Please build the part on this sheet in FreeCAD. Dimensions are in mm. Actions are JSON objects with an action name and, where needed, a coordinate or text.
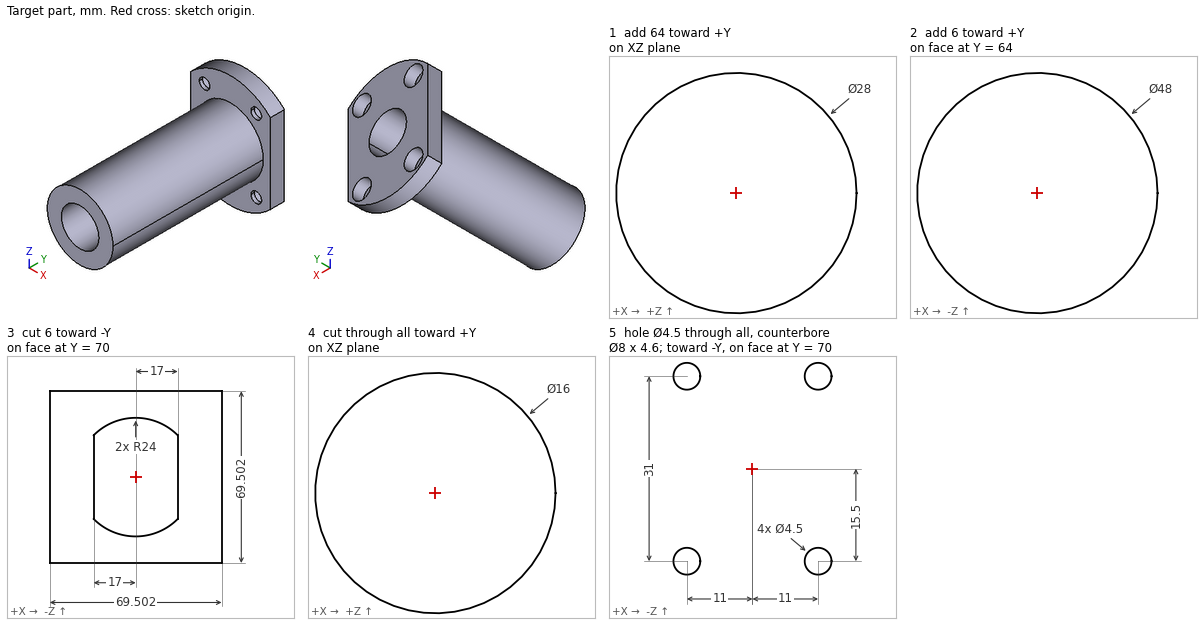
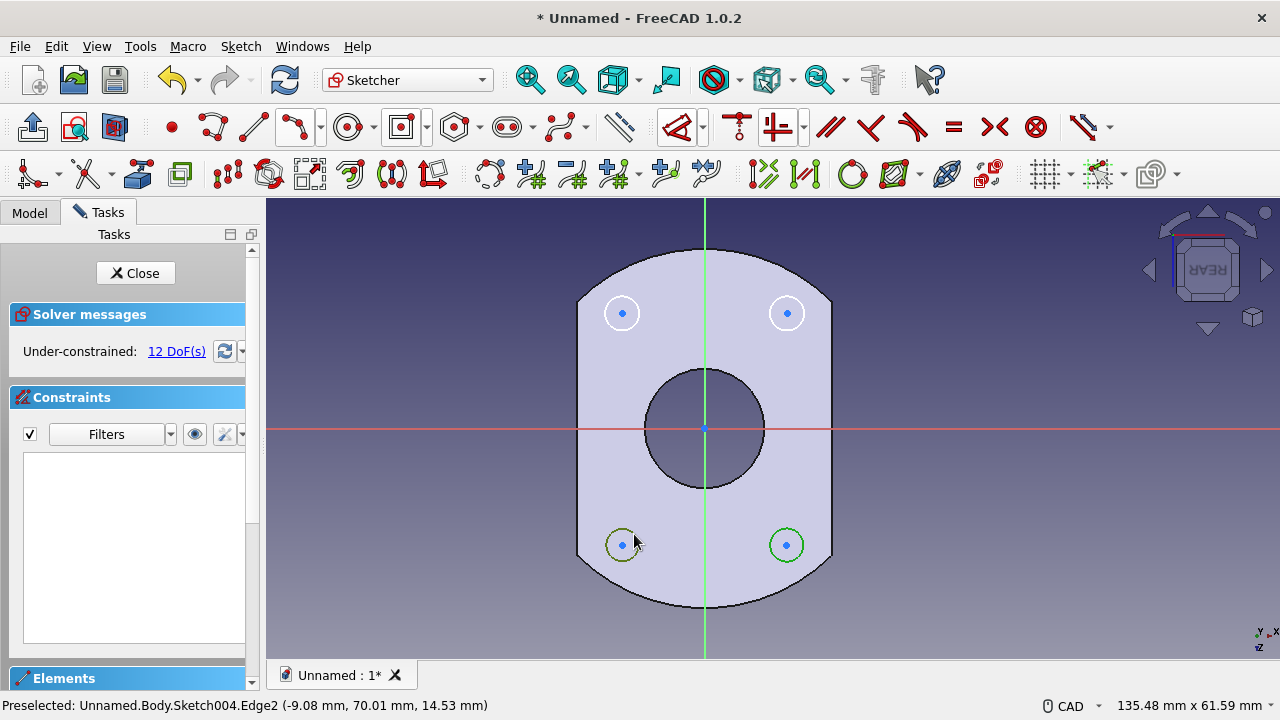
{"action": "left_click", "coordinate": [634, 301]}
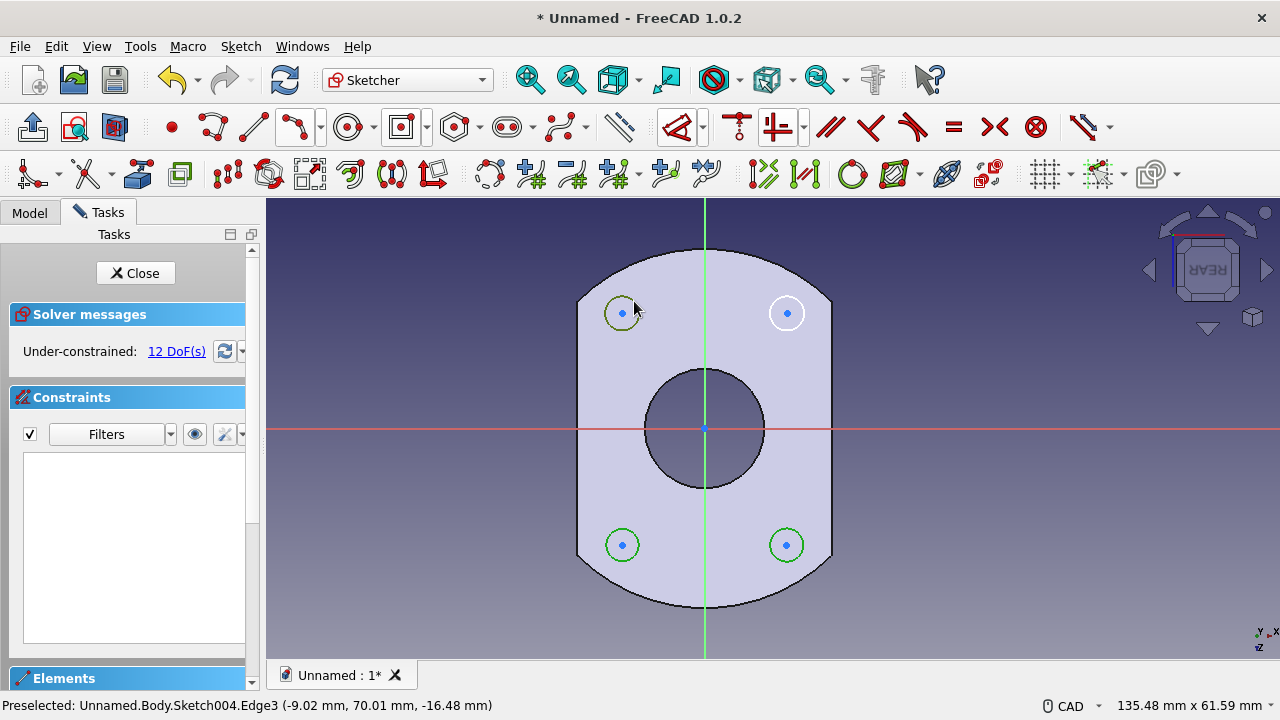
{"action": "left_click", "coordinate": [799, 301]}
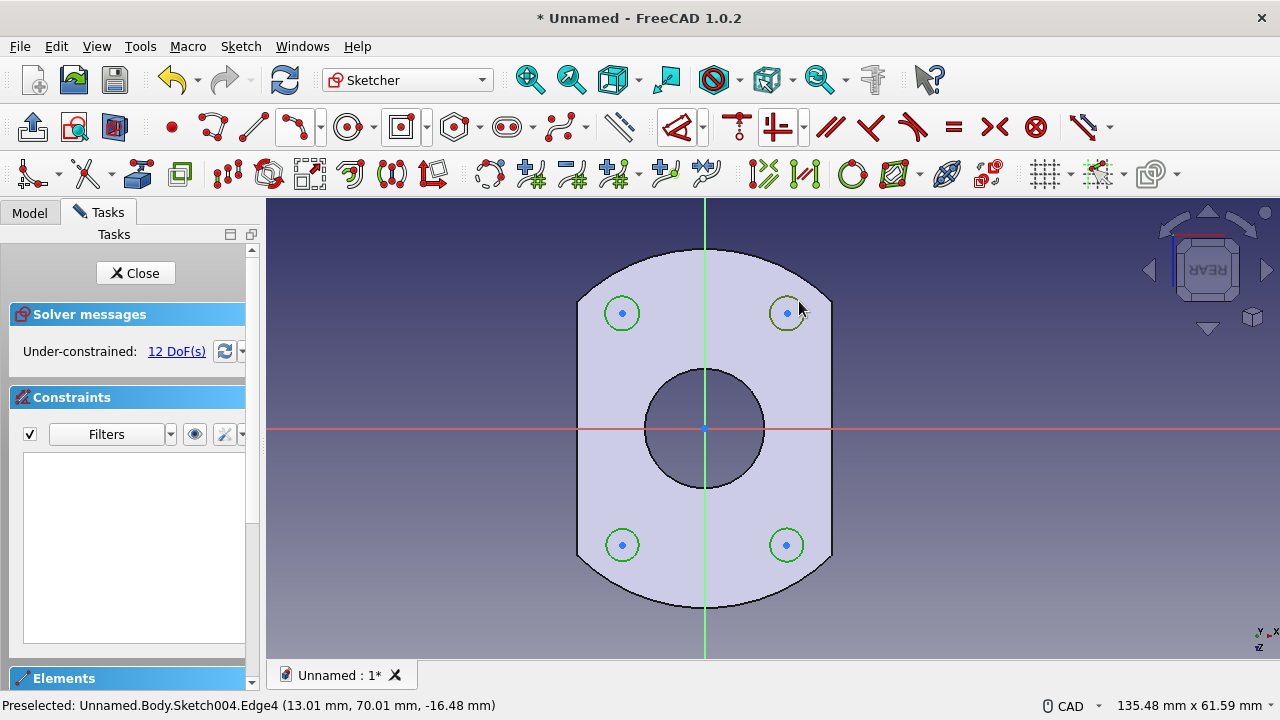
{"action": "left_click", "coordinate": [954, 128]}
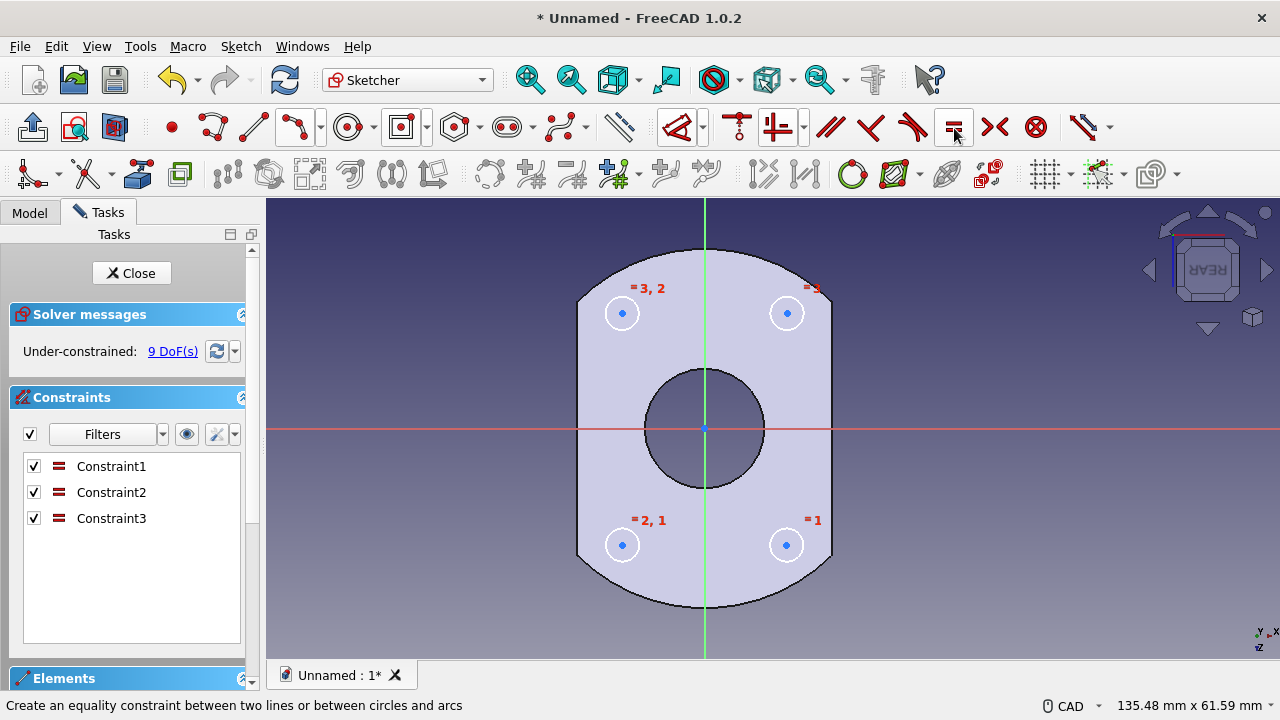
{"action": "left_click", "coordinate": [787, 545]}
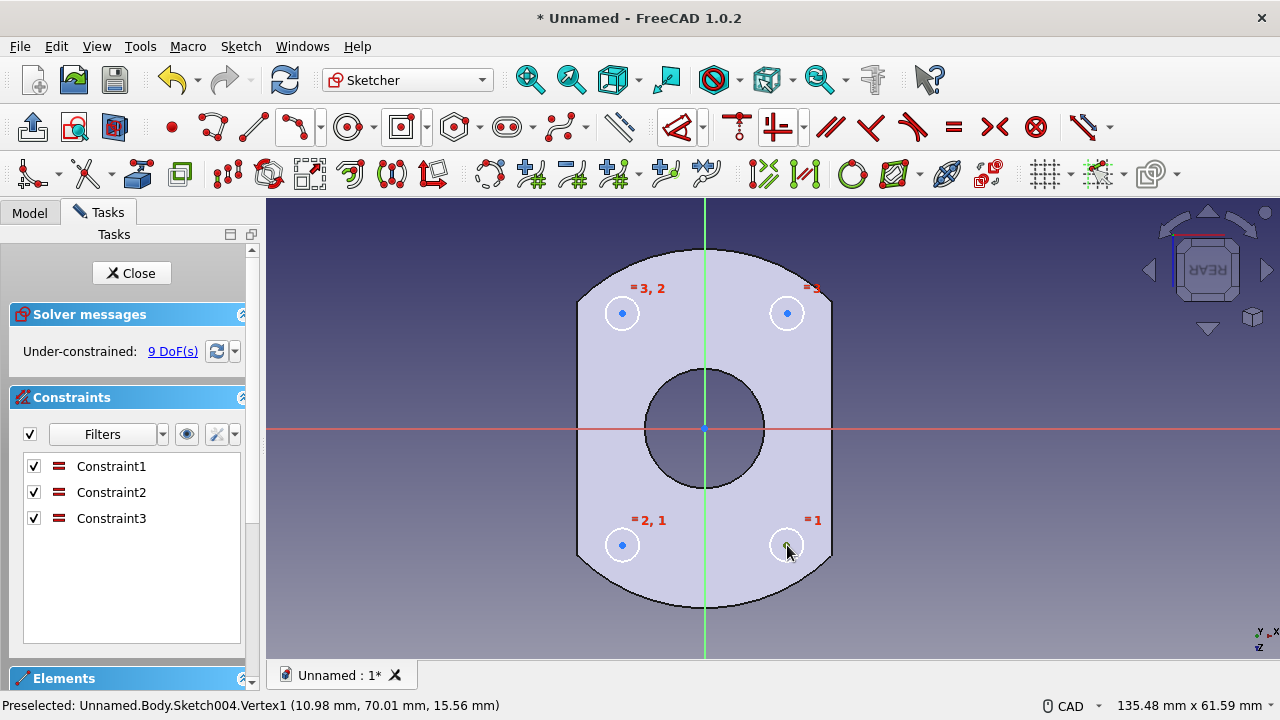
{"action": "left_click", "coordinate": [622, 545]}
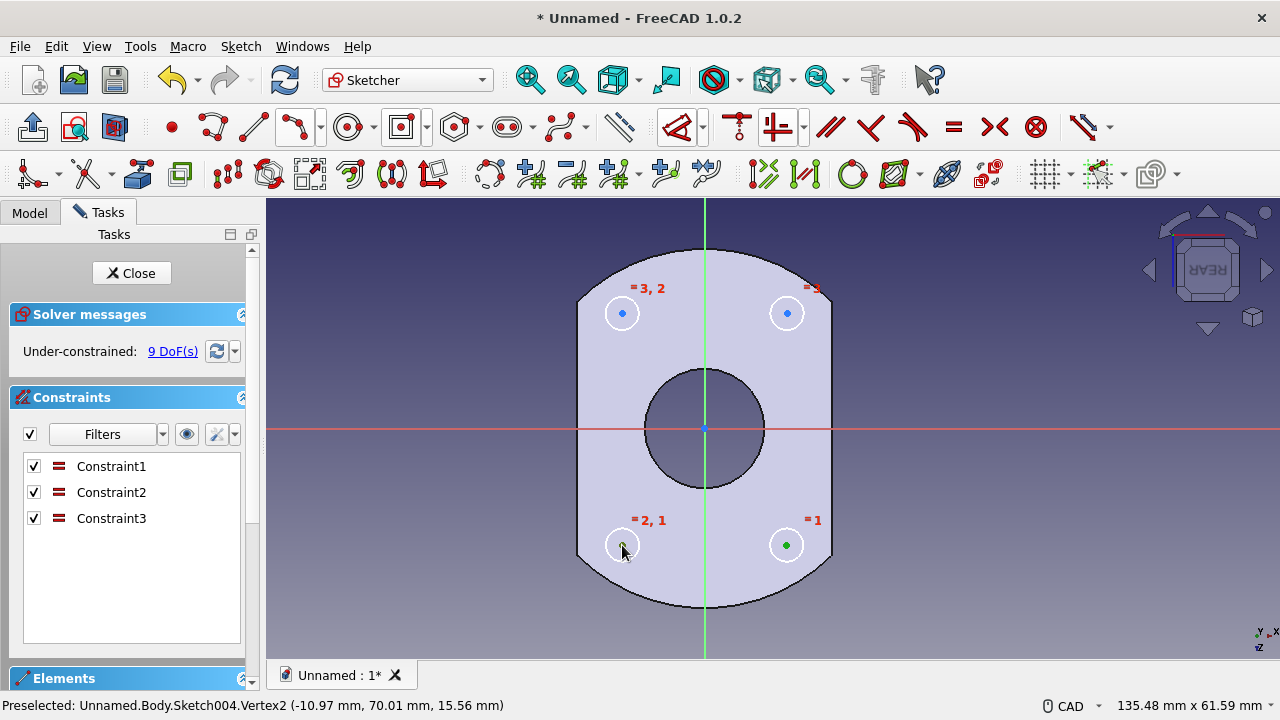
{"action": "key", "text": "h"}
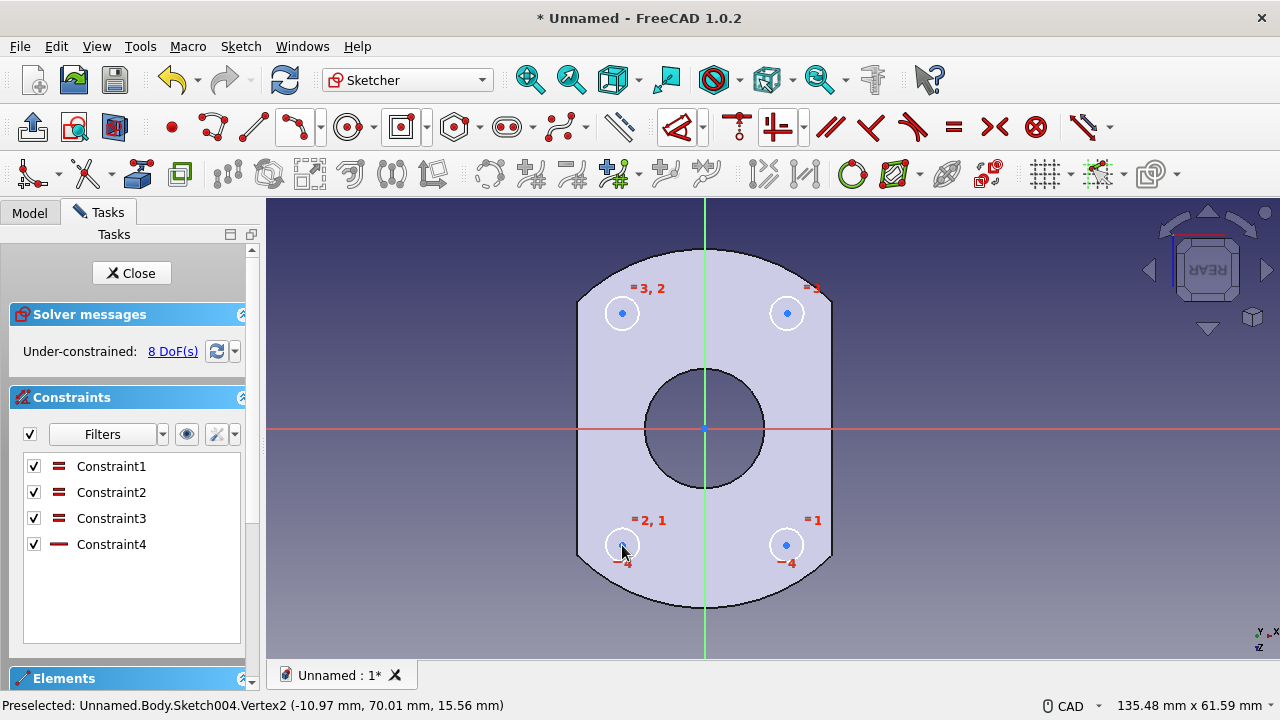
{"action": "left_click", "coordinate": [622, 545]}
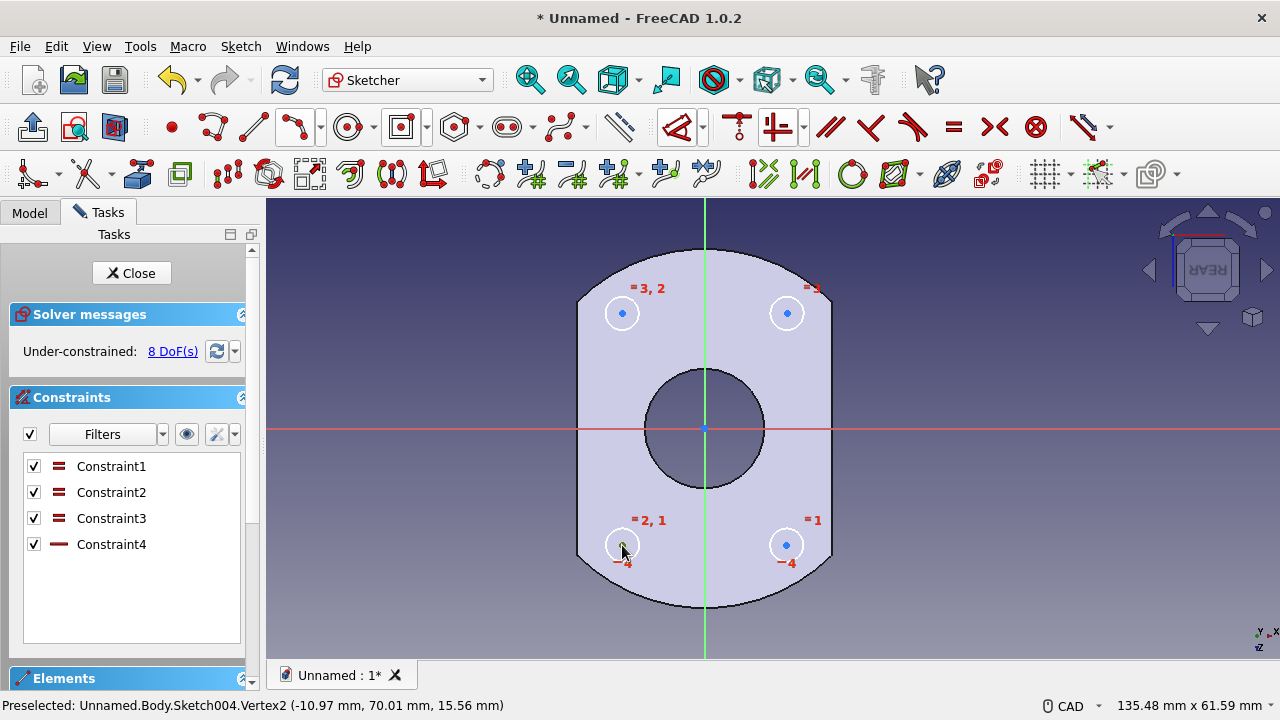
{"action": "left_click", "coordinate": [622, 313]}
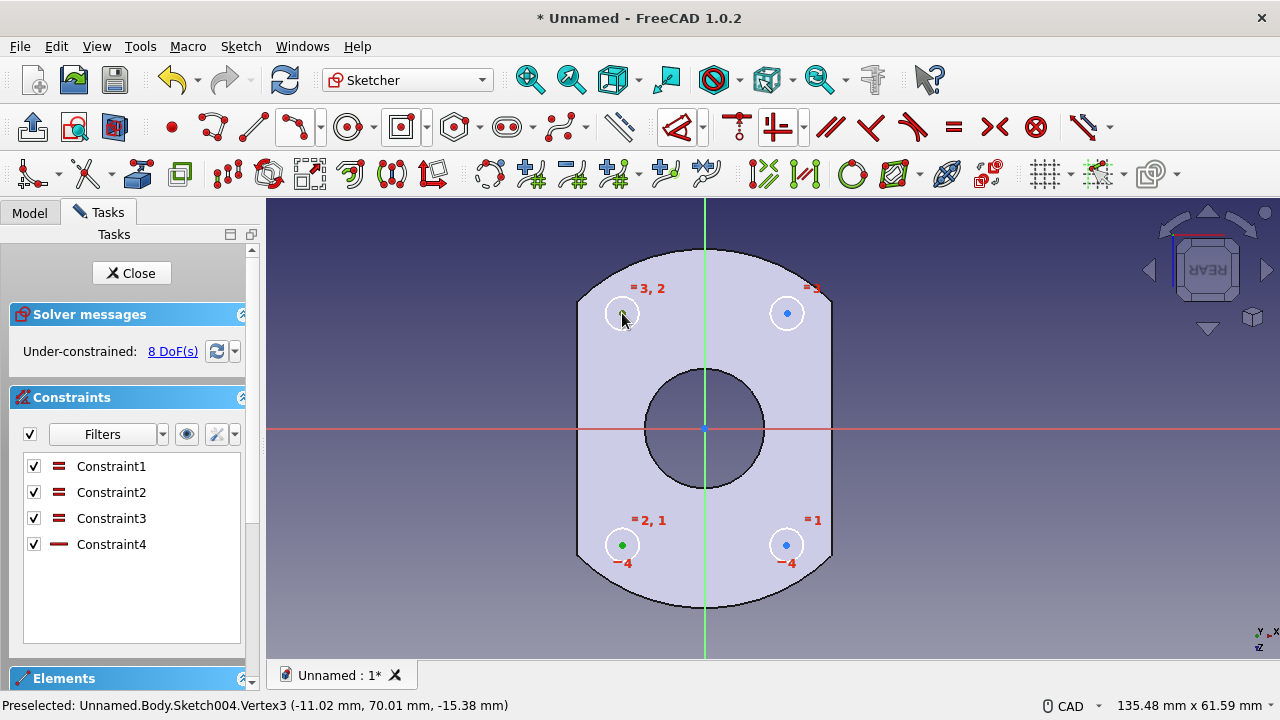
{"action": "key", "text": "v"}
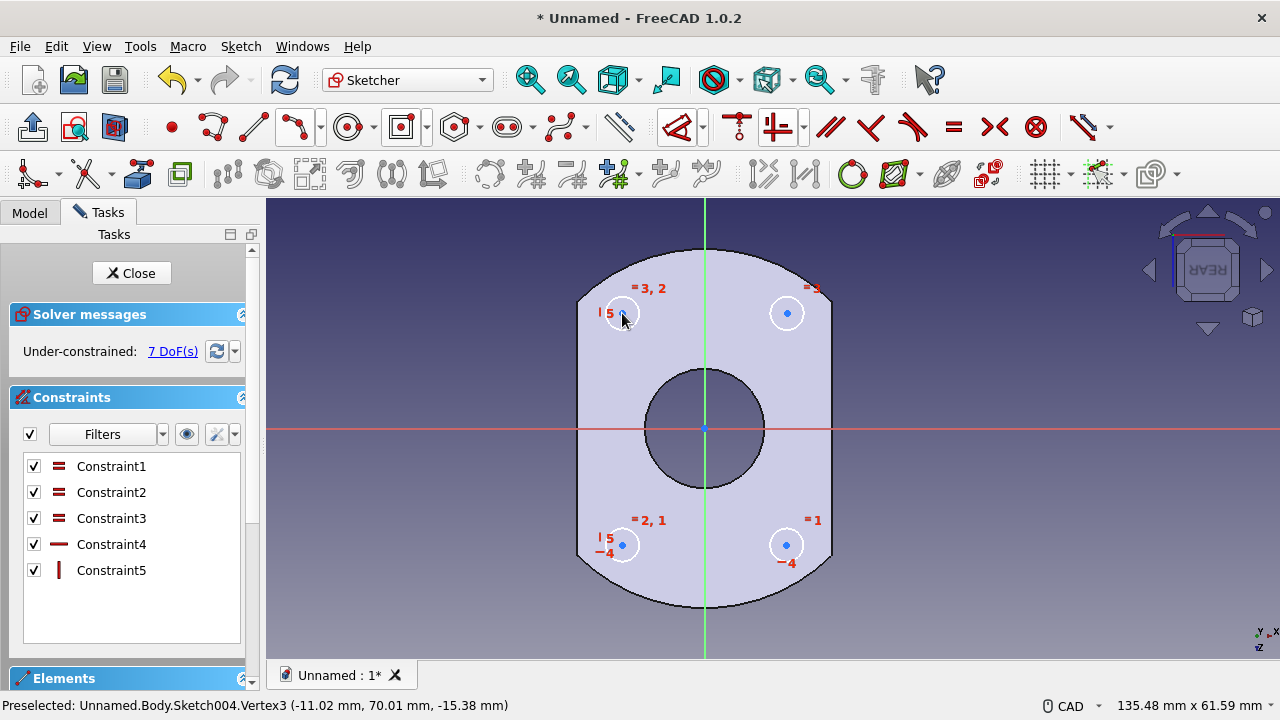
{"action": "left_click", "coordinate": [787, 545]}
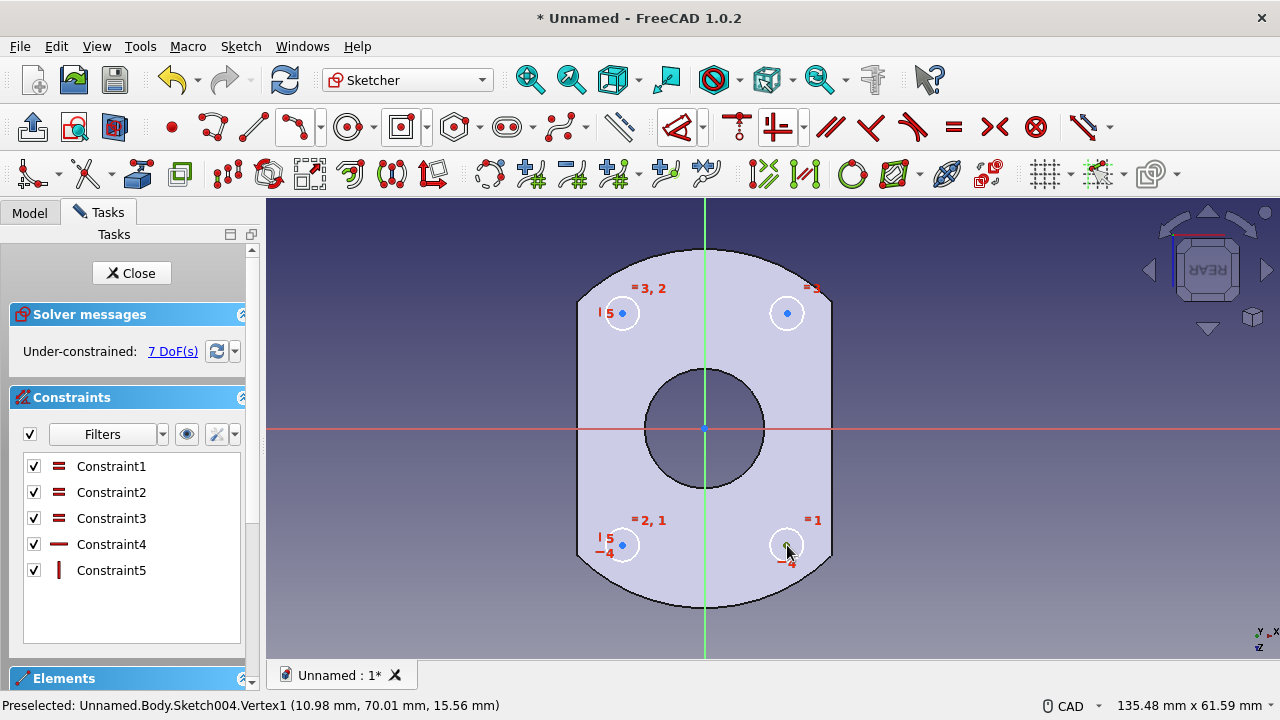
{"action": "left_click", "coordinate": [787, 313]}